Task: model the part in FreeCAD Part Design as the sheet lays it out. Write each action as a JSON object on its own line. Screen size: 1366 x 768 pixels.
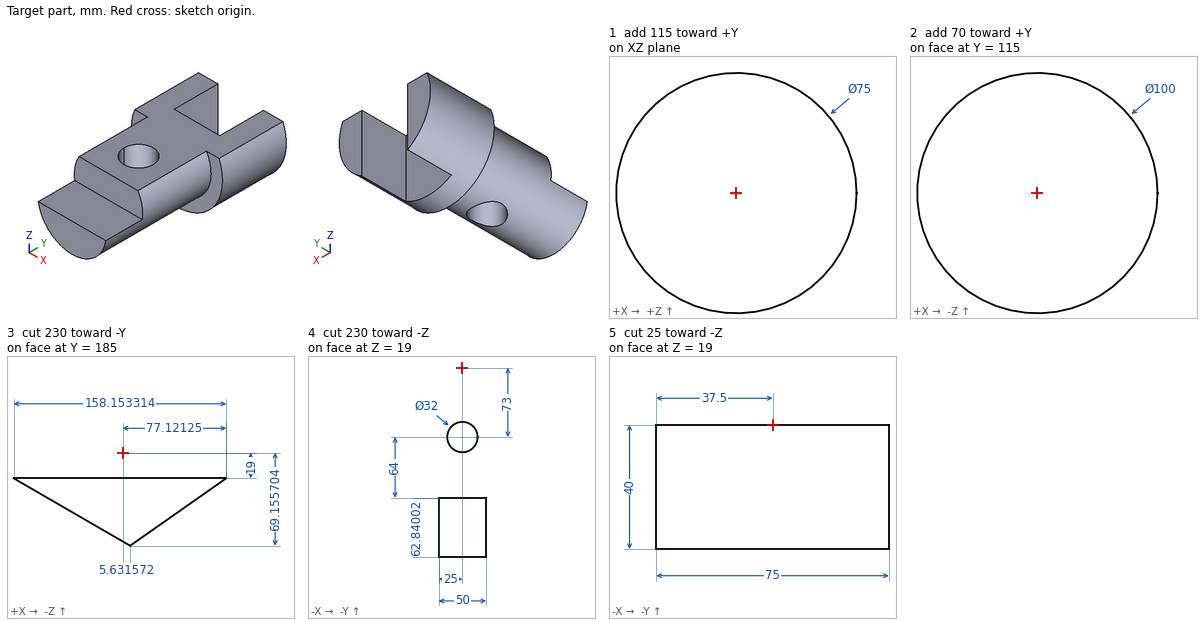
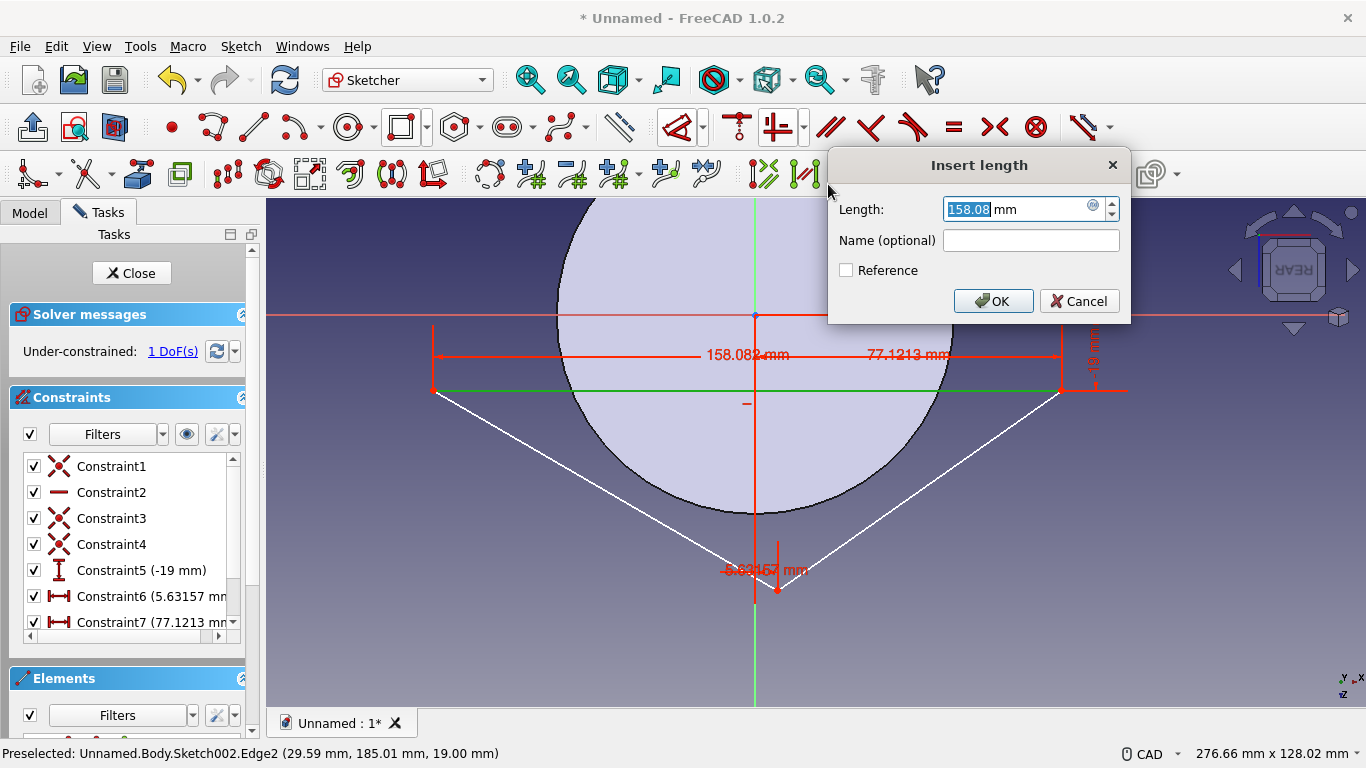
{"action": "type", "text": "158.153314"}
{"action": "key", "text": "Return"}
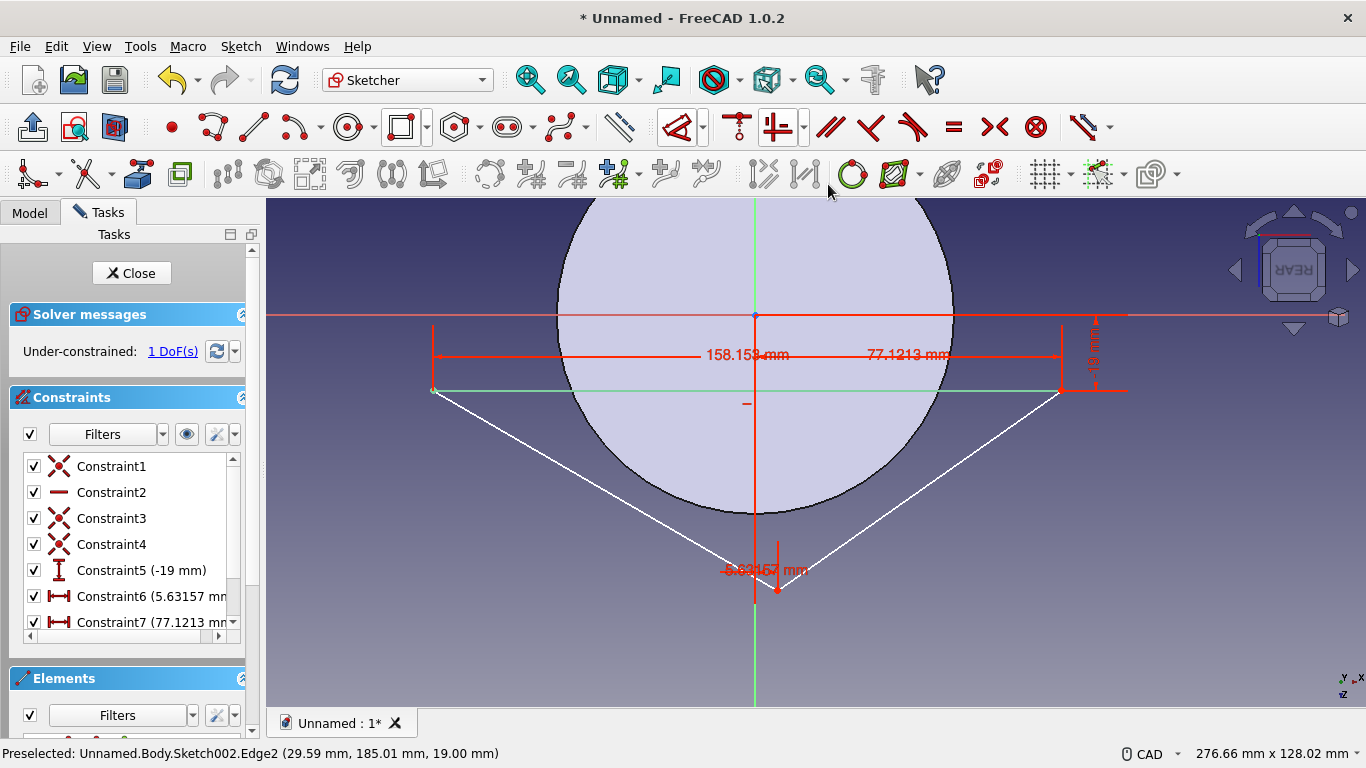
{"action": "left_click", "coordinate": [778, 591]}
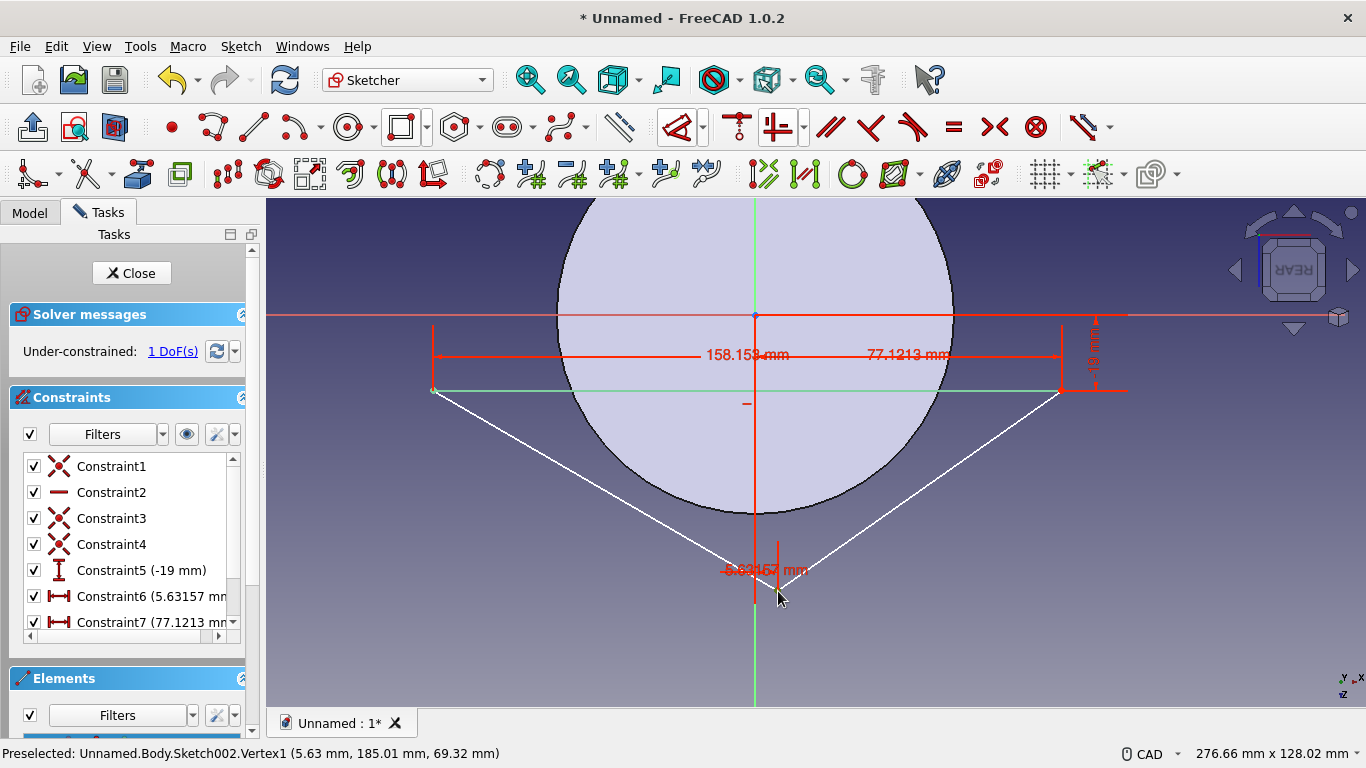
{"action": "left_click", "coordinate": [702, 128]}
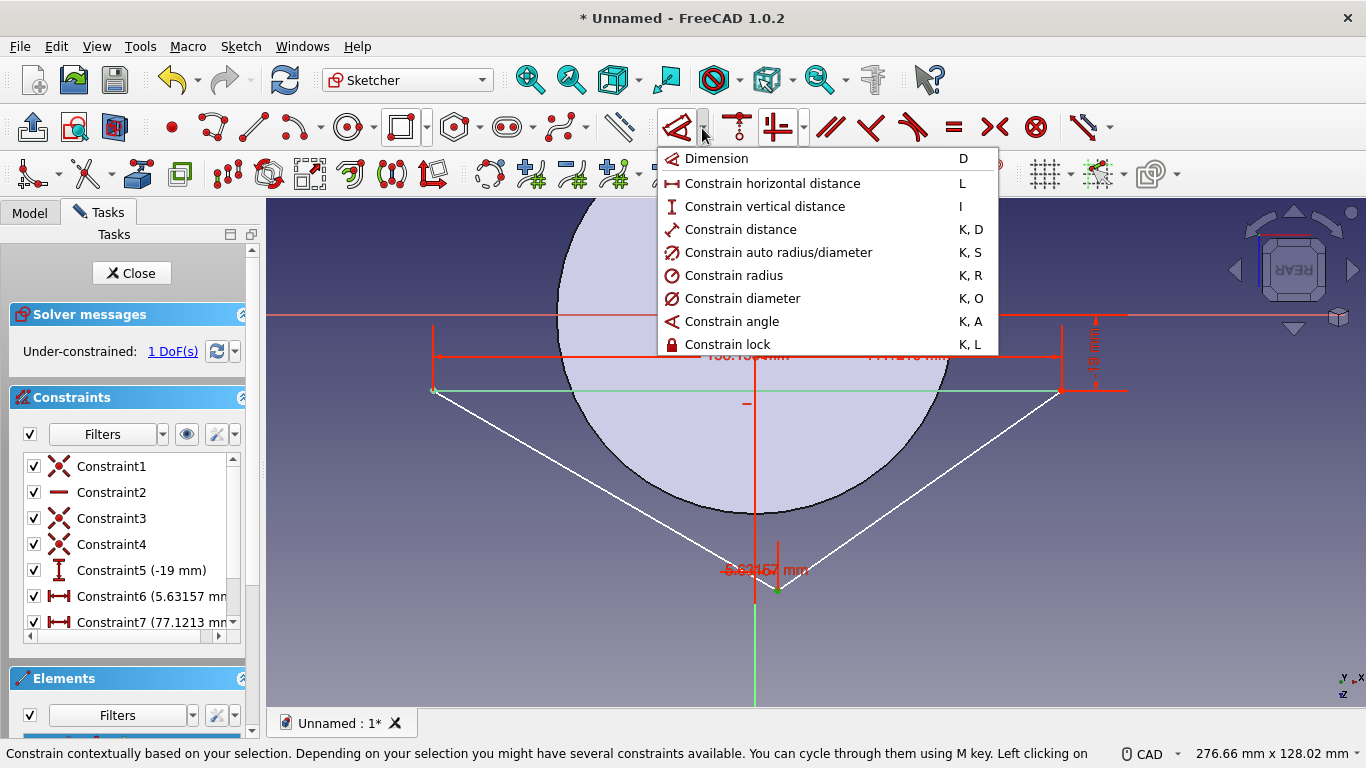
{"action": "left_click", "coordinate": [828, 206]}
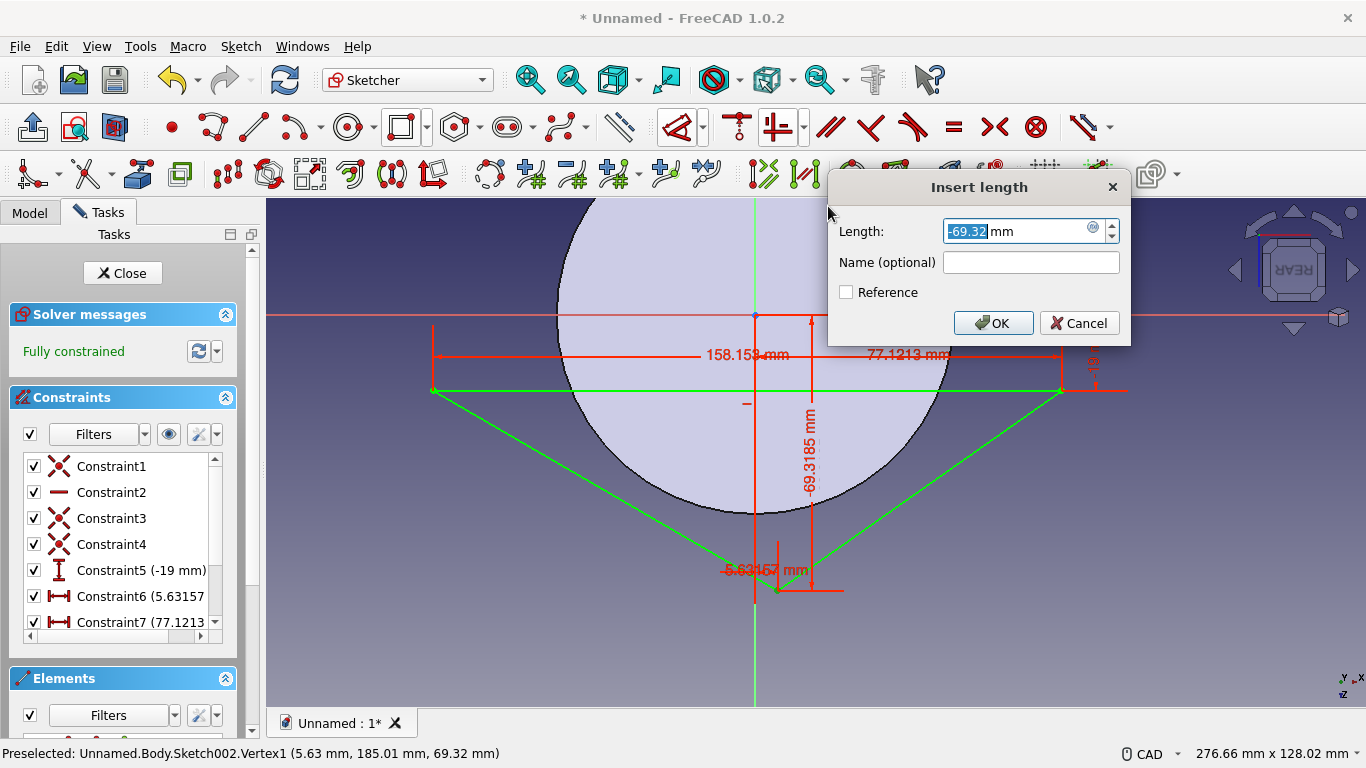
{"action": "type", "text": "-69.155704"}
{"action": "key", "text": "Return"}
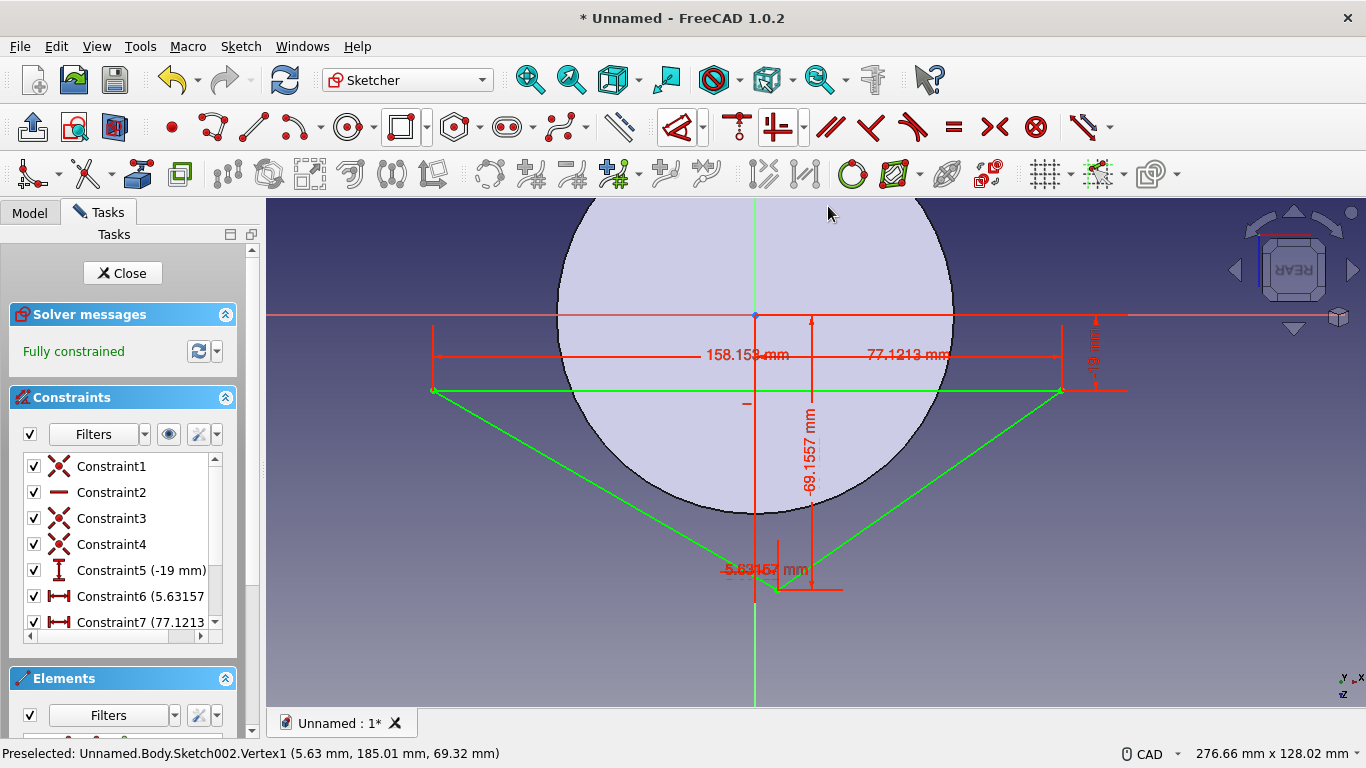
{"action": "left_click", "coordinate": [123, 273]}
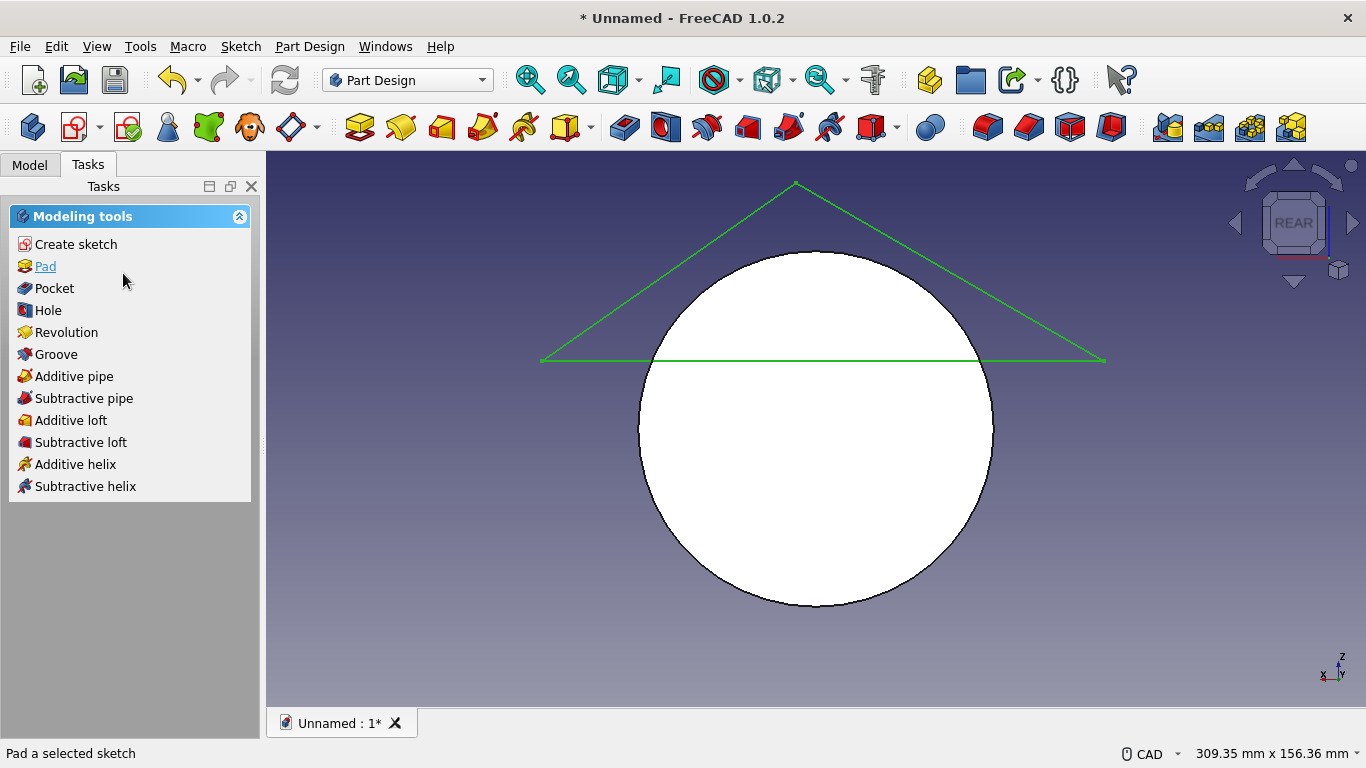
{"action": "left_click", "coordinate": [625, 128]}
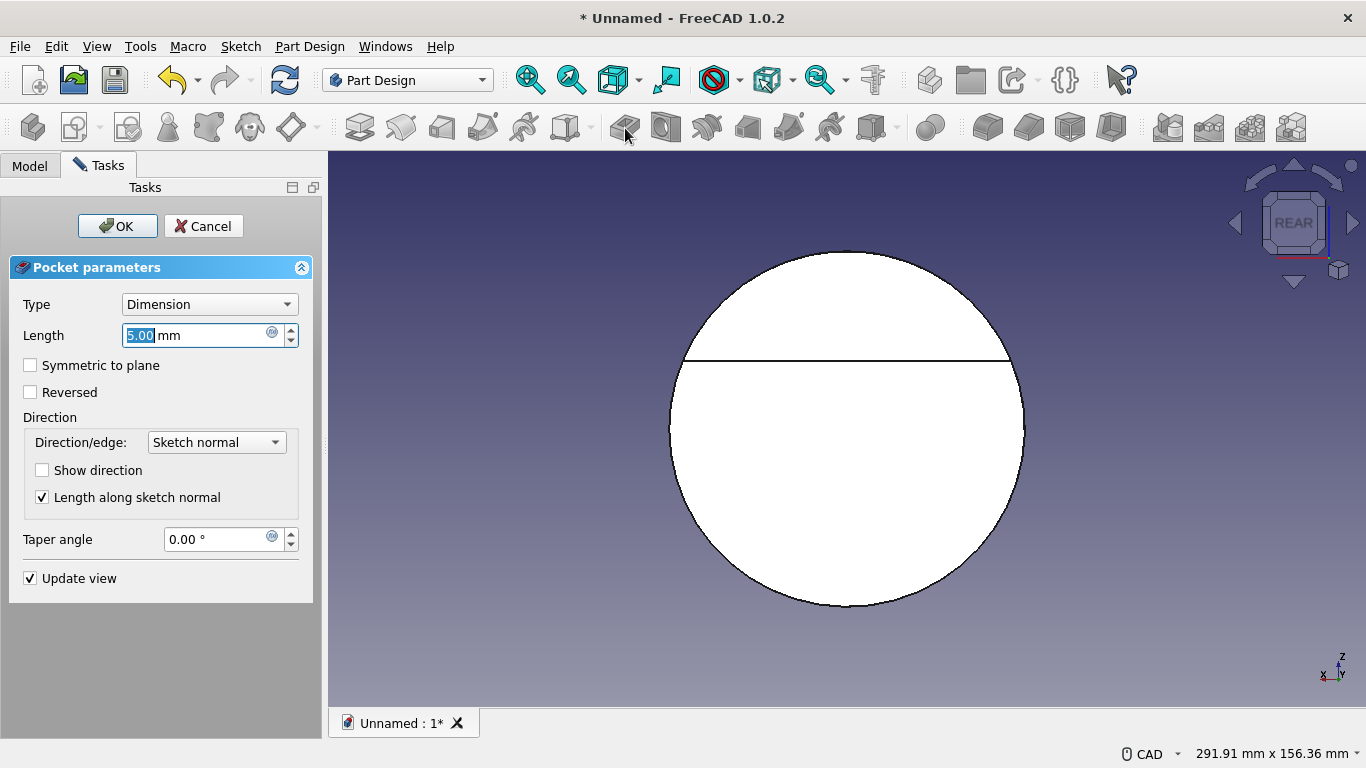
{"action": "type", "text": "230"}
{"action": "key", "text": "Tab"}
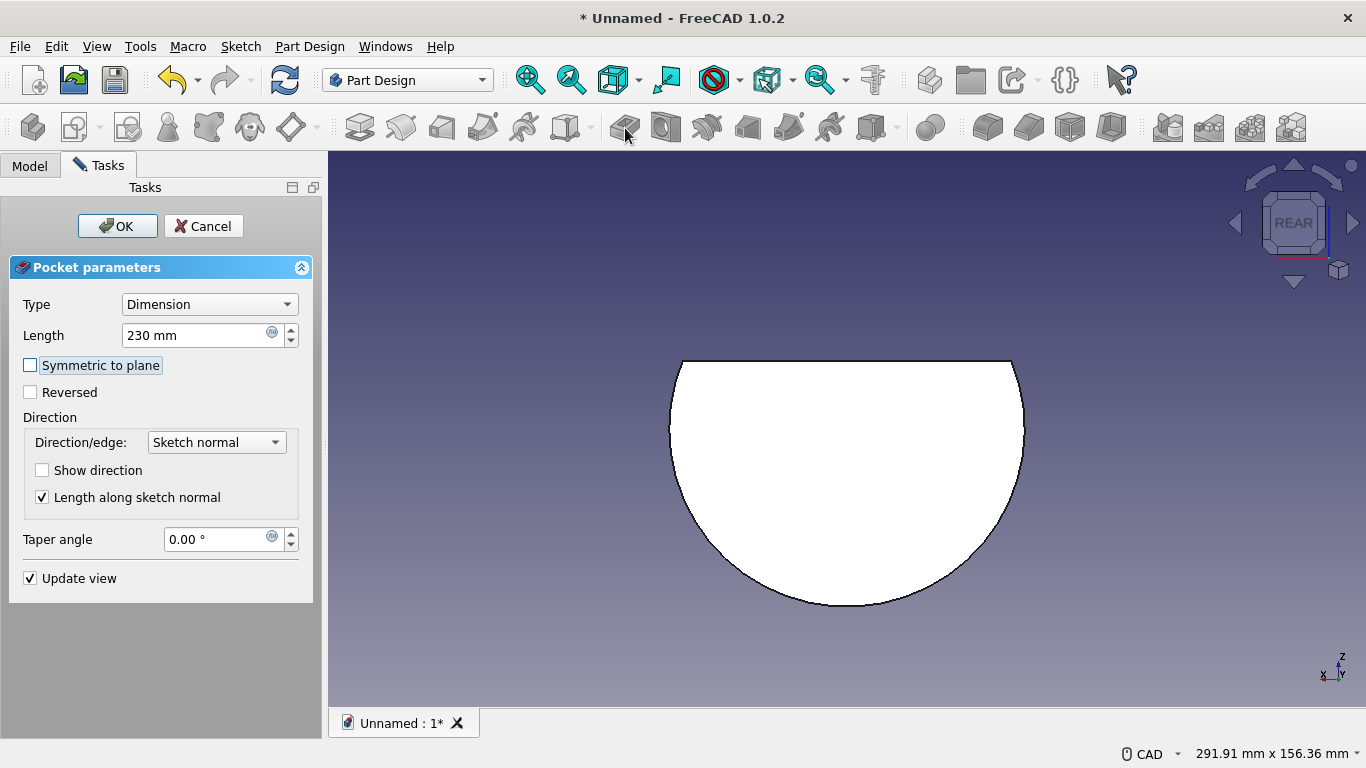
{"action": "left_click", "coordinate": [118, 226]}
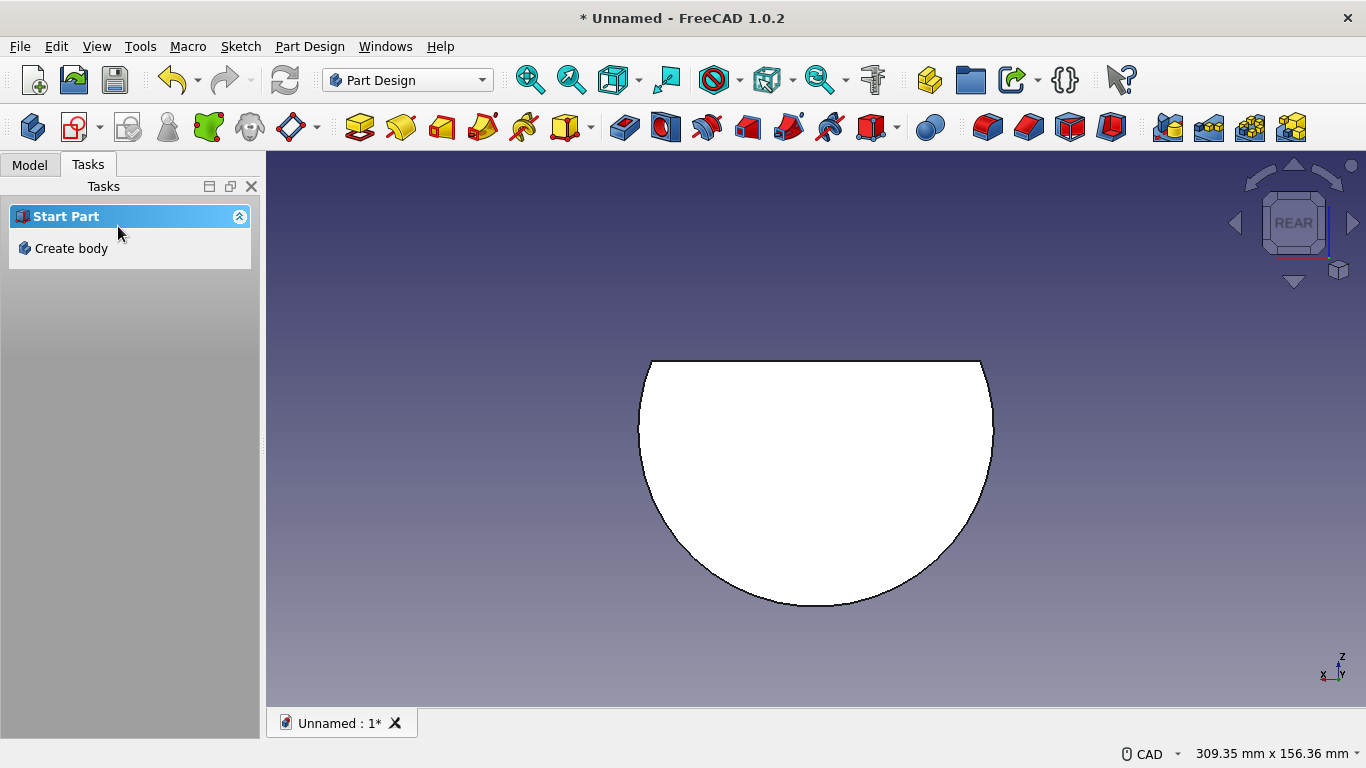
{"action": "left_click", "coordinate": [531, 80]}